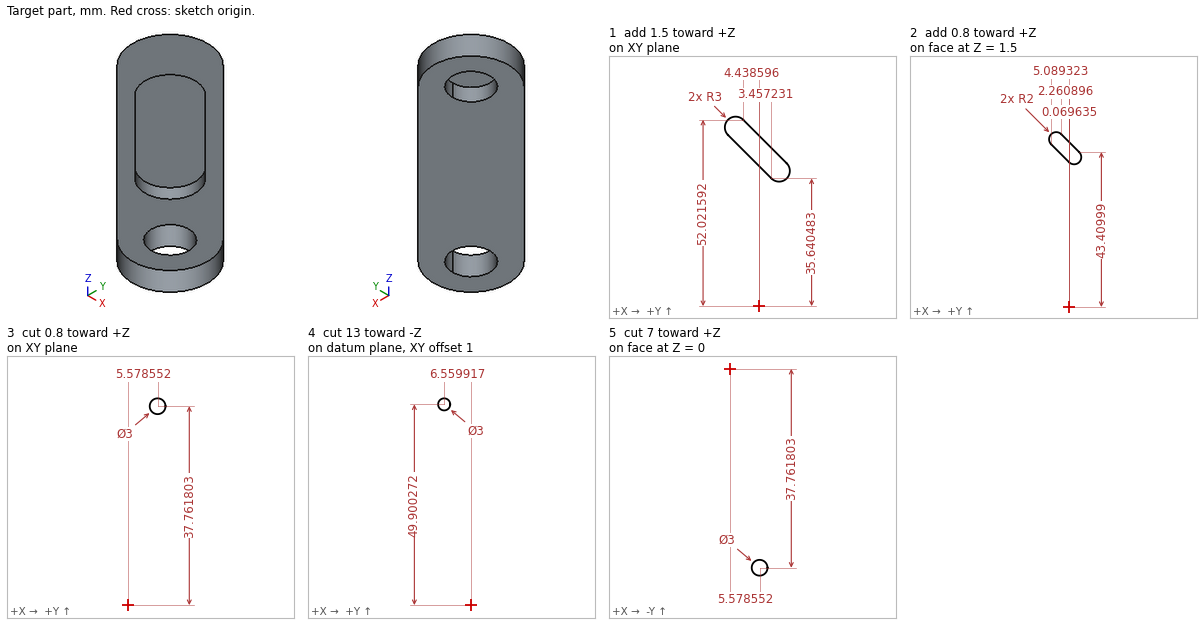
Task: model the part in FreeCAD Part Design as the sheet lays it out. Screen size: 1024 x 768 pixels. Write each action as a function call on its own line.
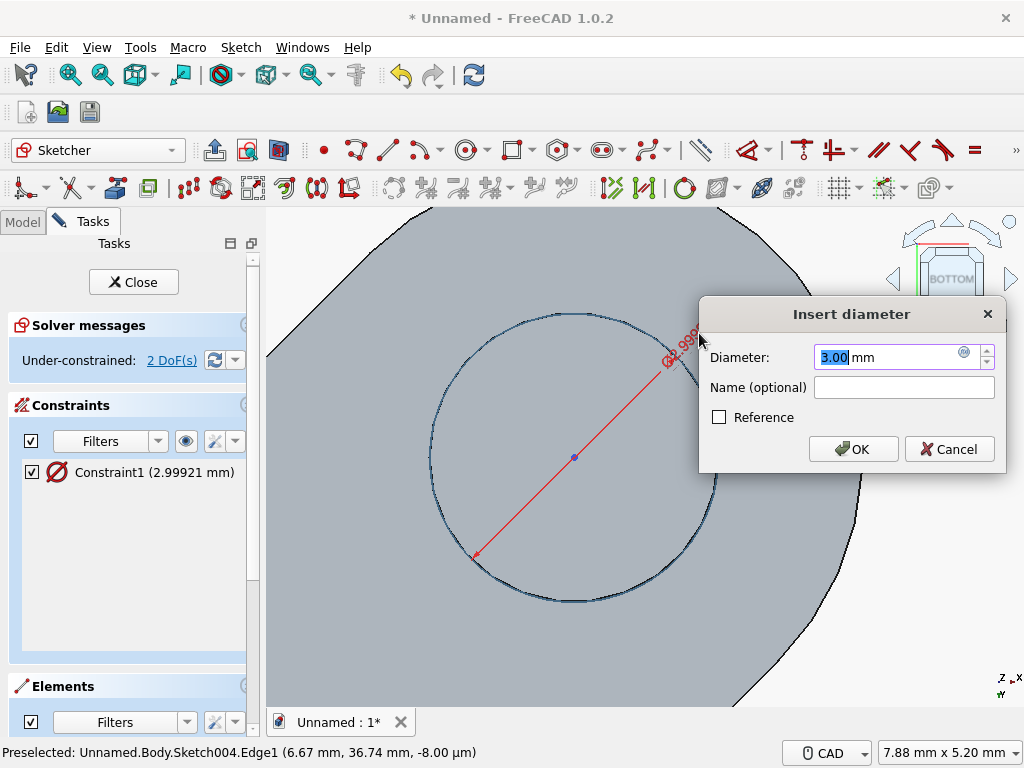
text(3)
key(Return)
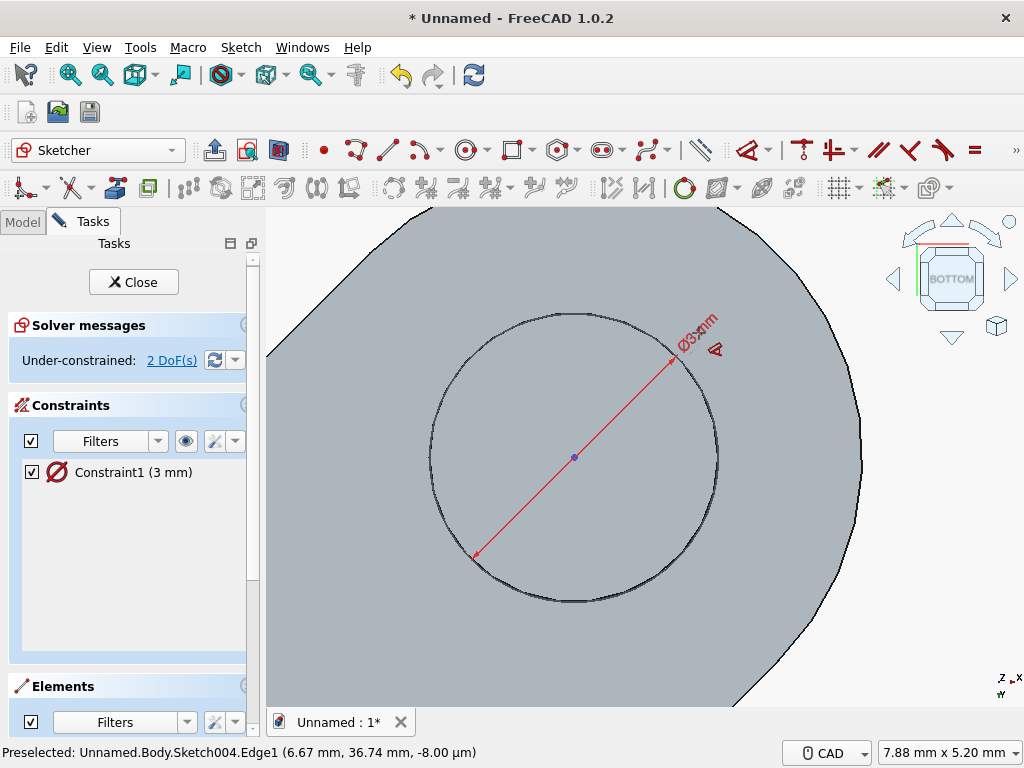
click(574, 458)
click(370, 492)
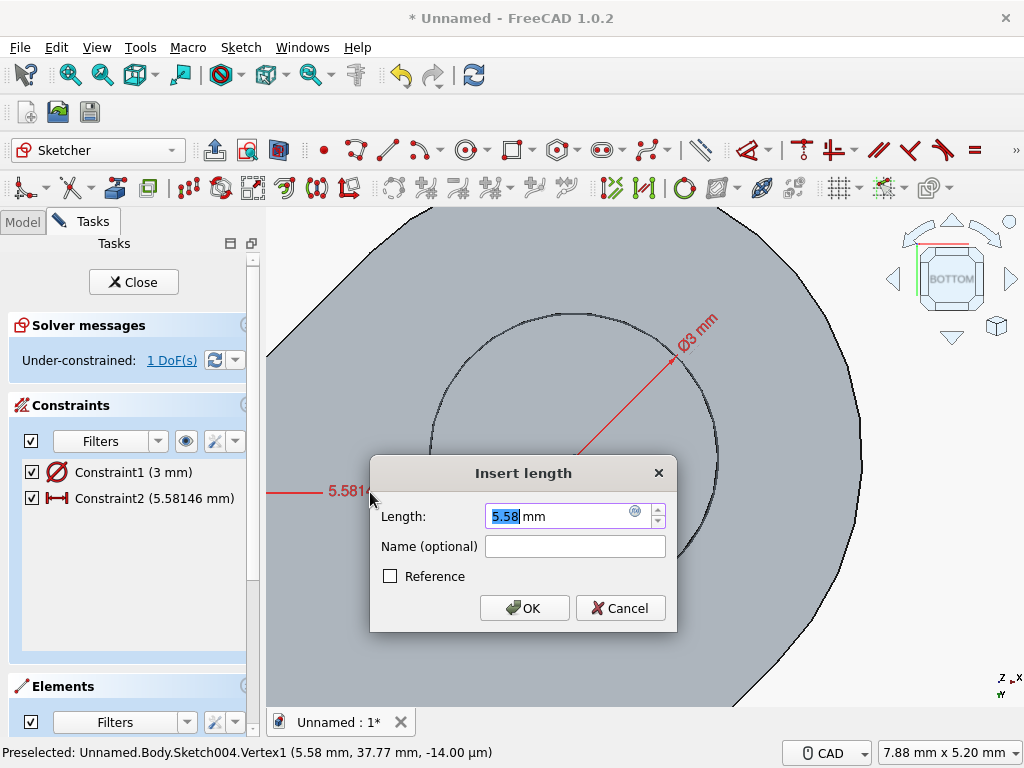
text(5.578552)
key(Return)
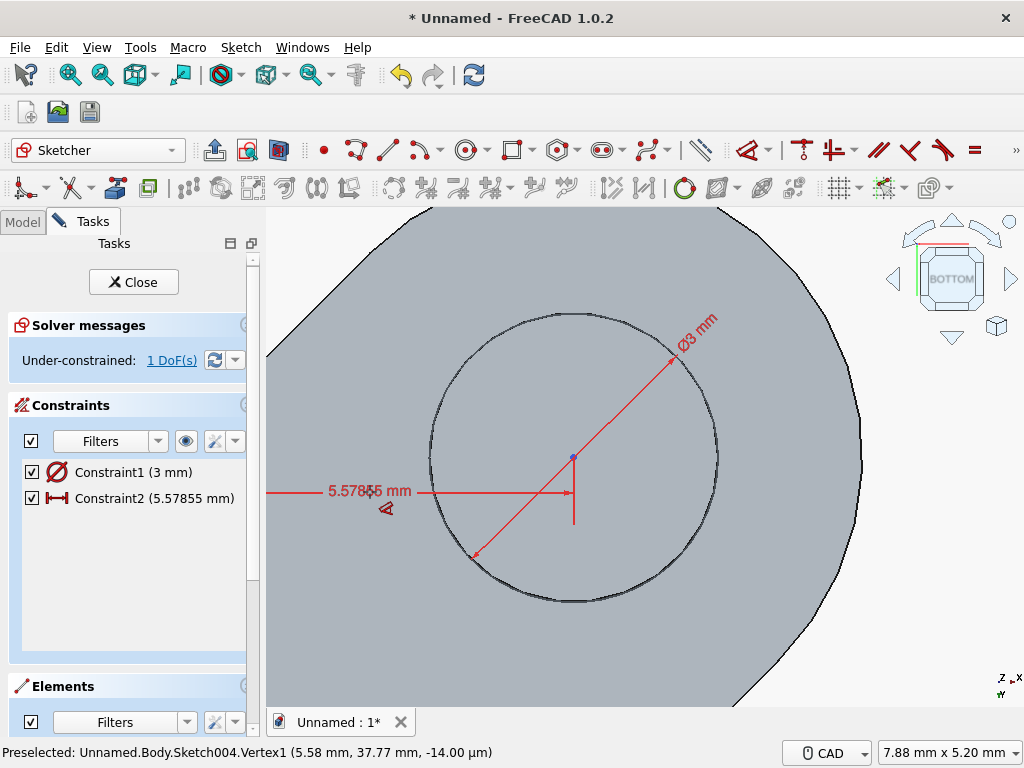
click(574, 458)
click(608, 346)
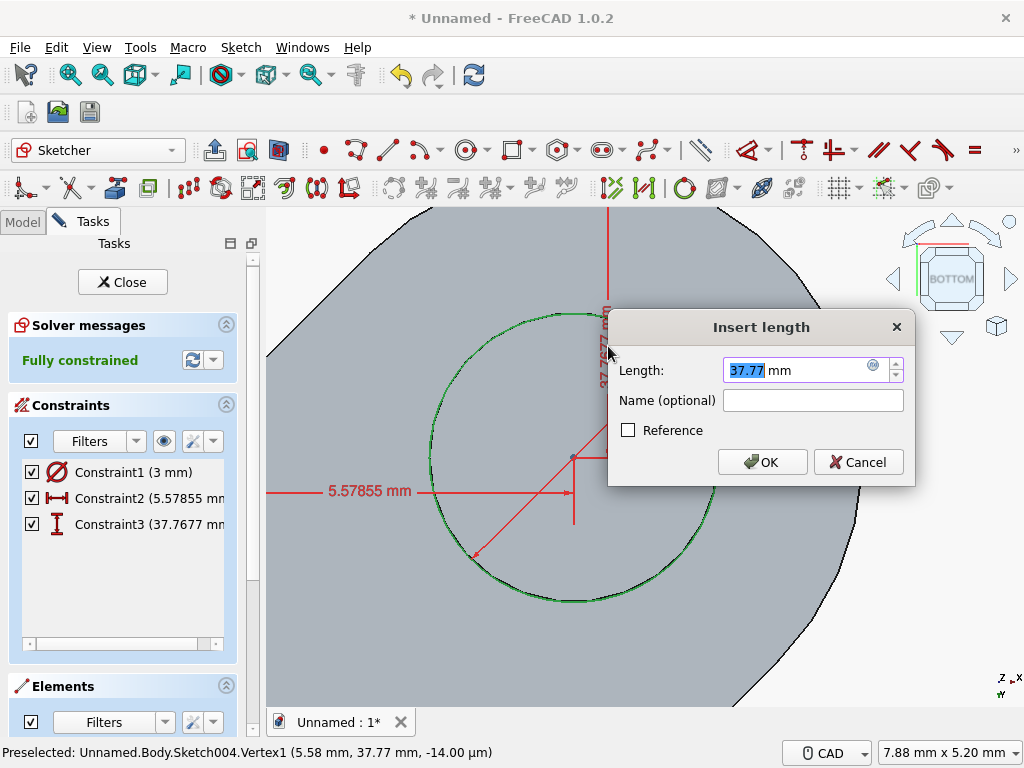
text(37.761803)
key(Return)
key(Escape)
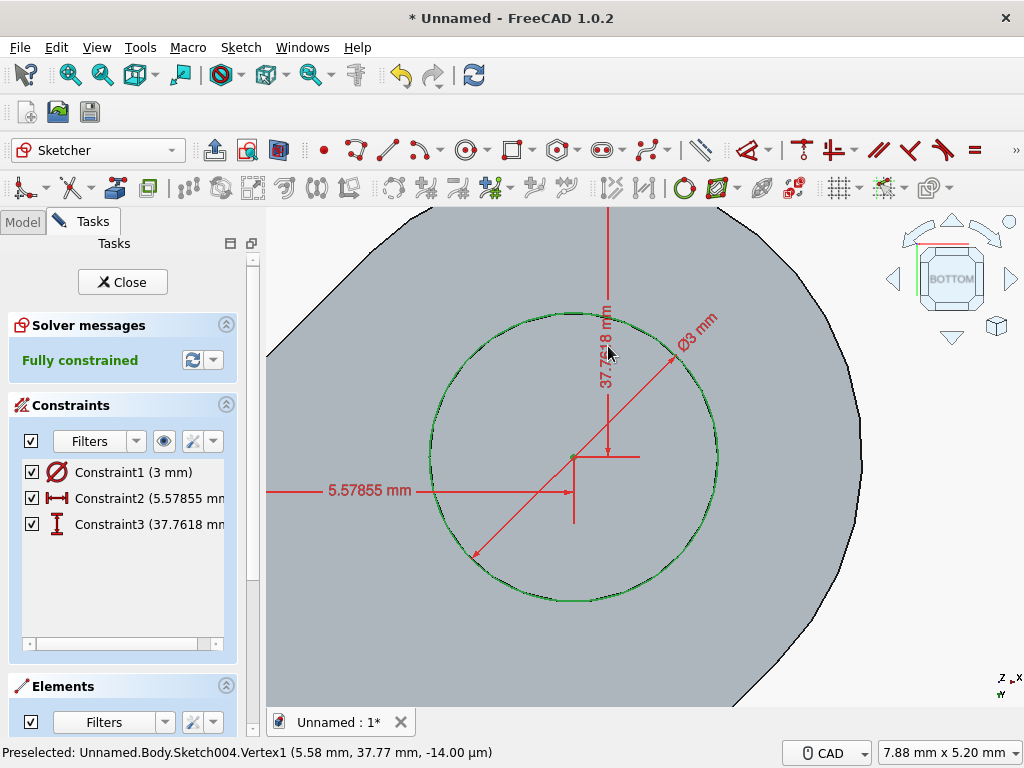
click(123, 282)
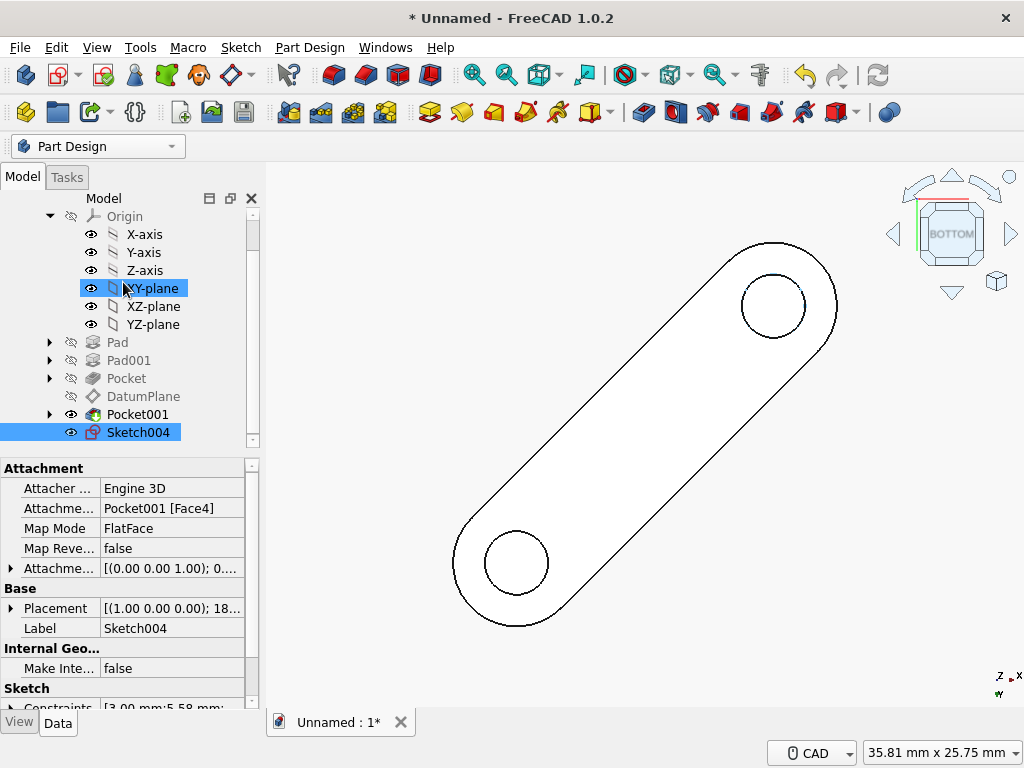
click(644, 112)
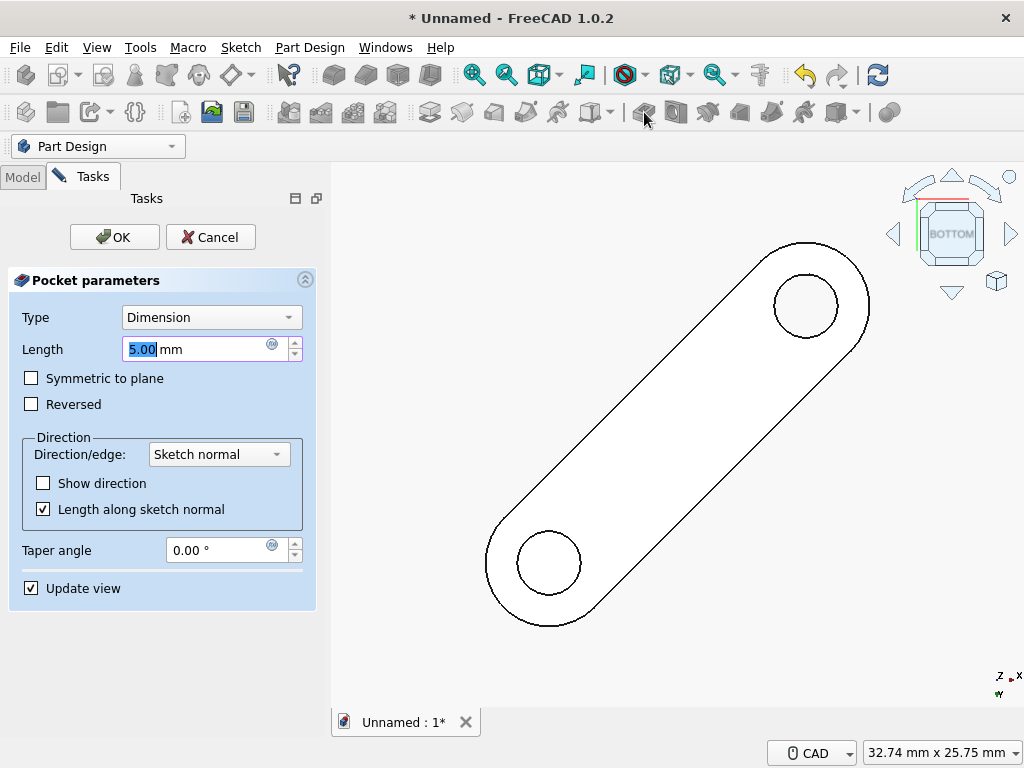
text(7)
key(Tab)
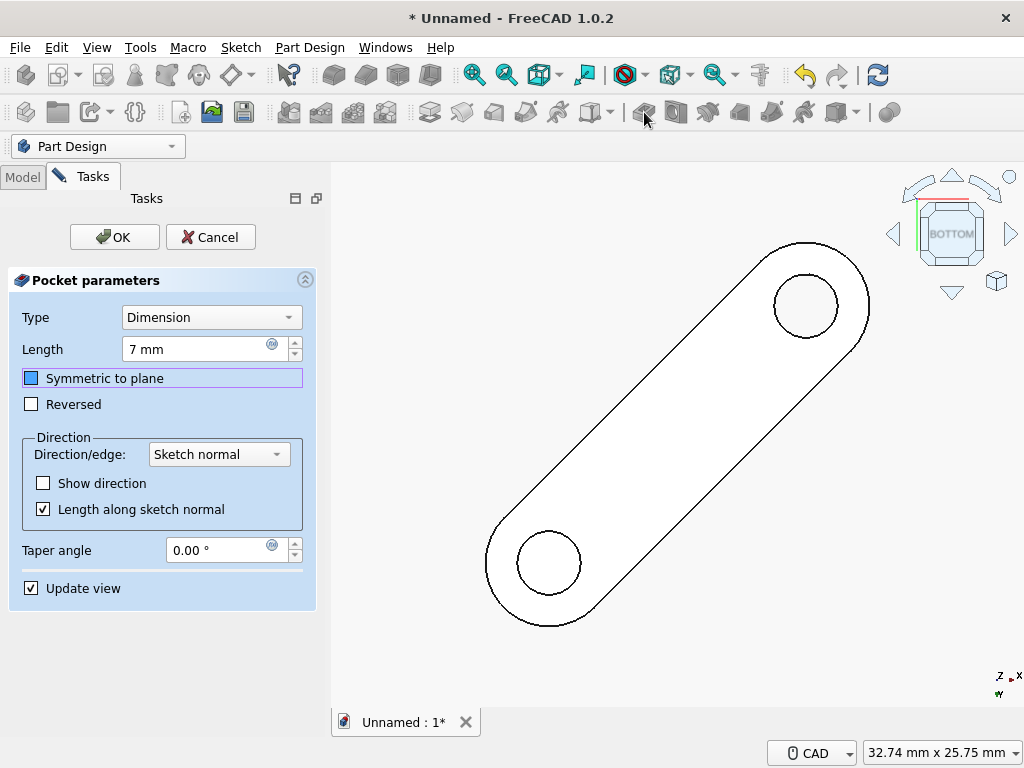
click(115, 237)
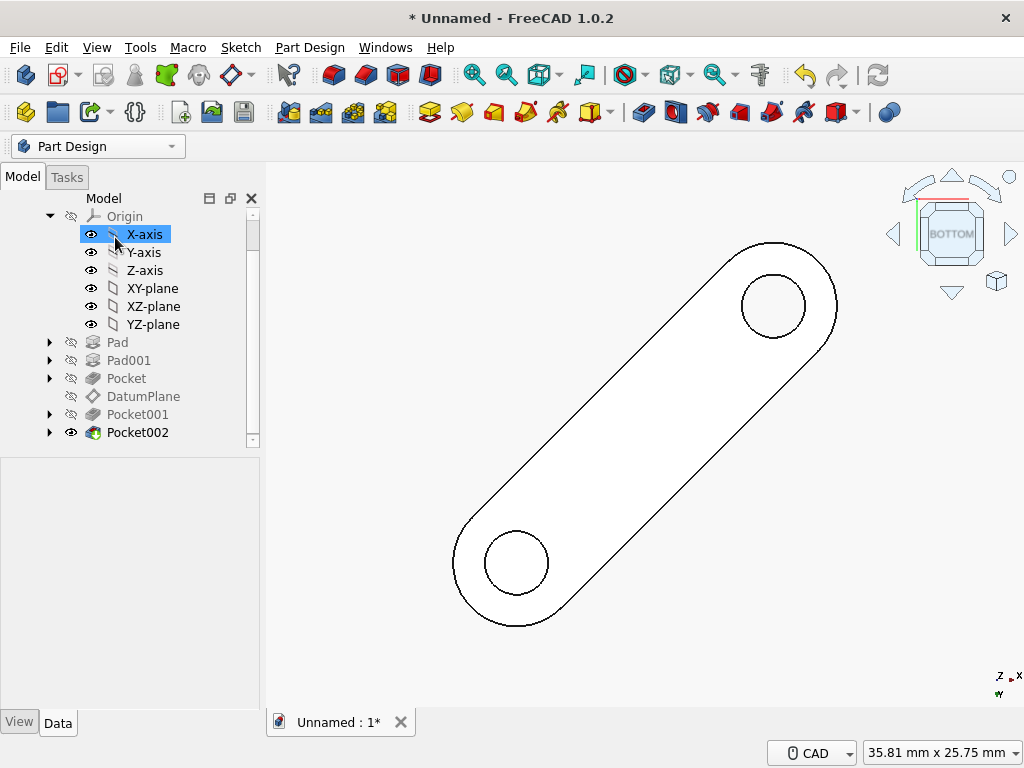
key(0)